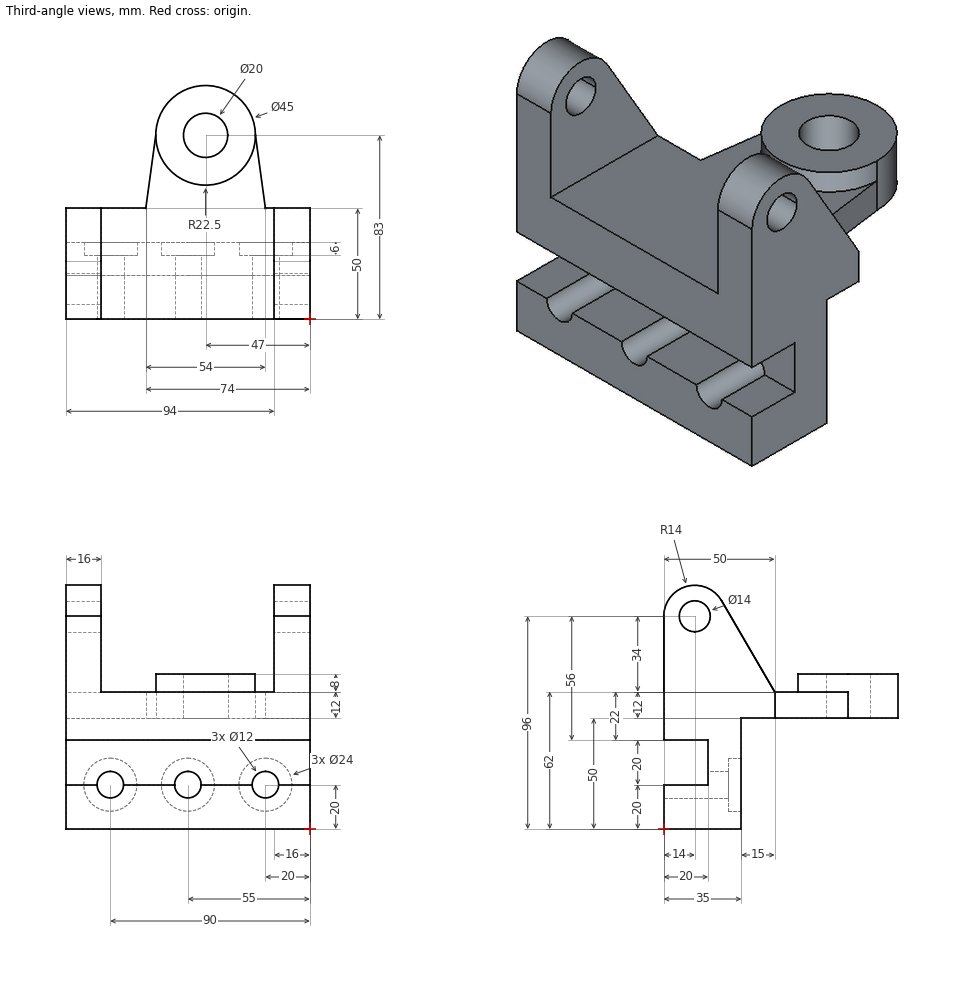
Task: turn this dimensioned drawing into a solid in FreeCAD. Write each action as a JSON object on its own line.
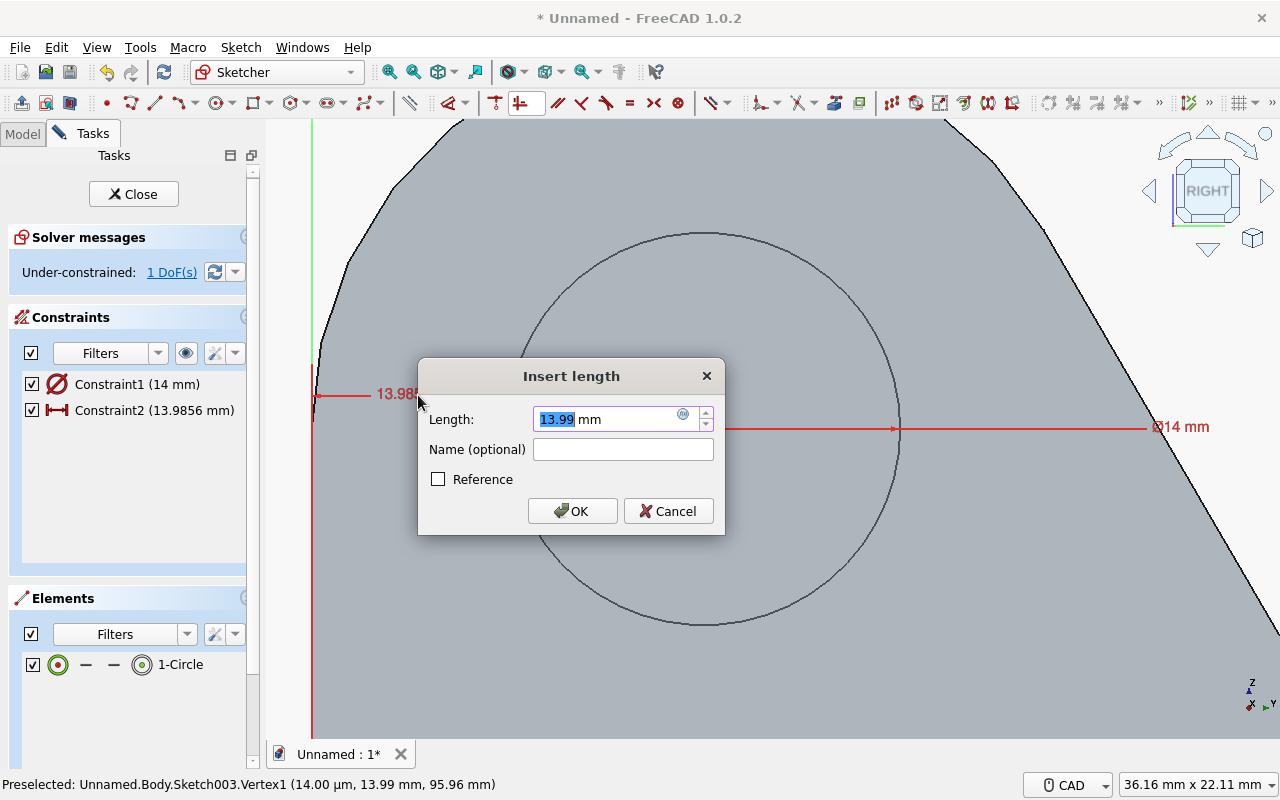
{"action": "type", "text": "14"}
{"action": "key", "text": "Return"}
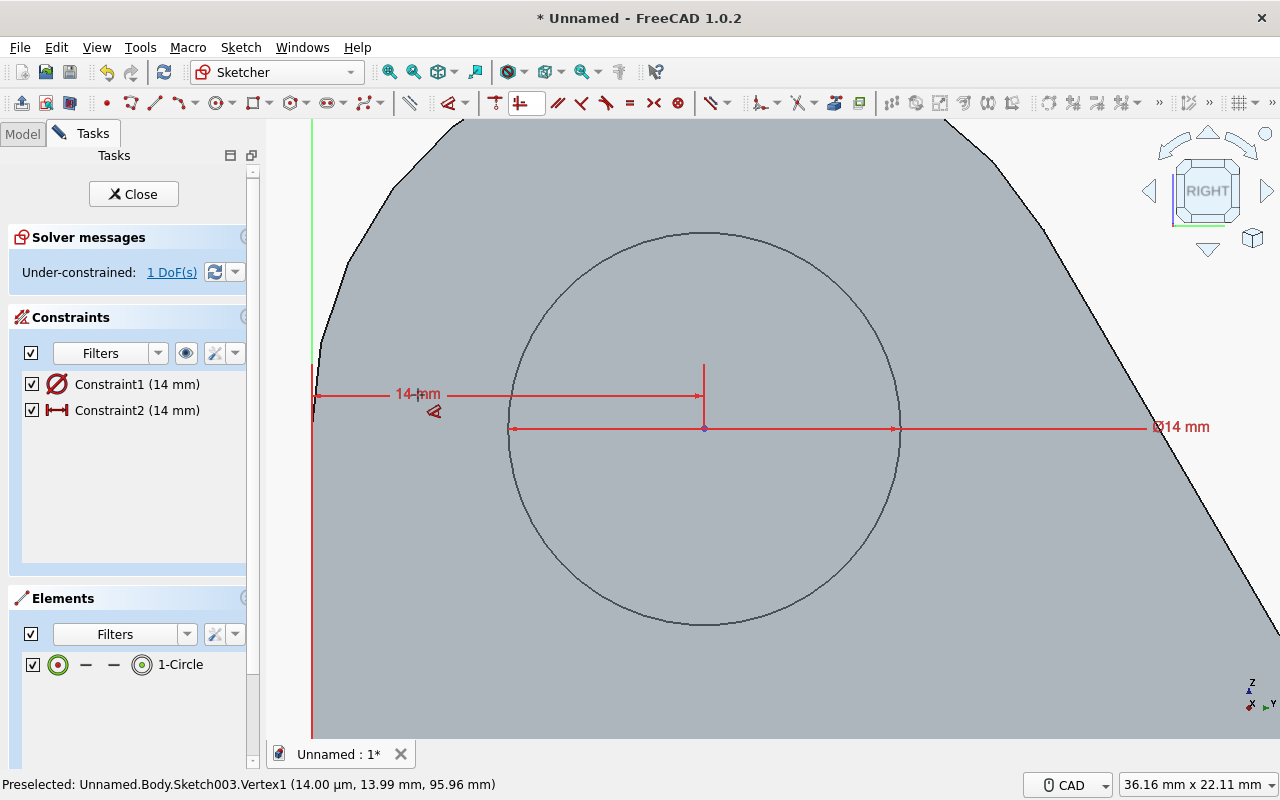
{"action": "left_click", "coordinate": [704, 429]}
{"action": "left_click", "coordinate": [738, 570]}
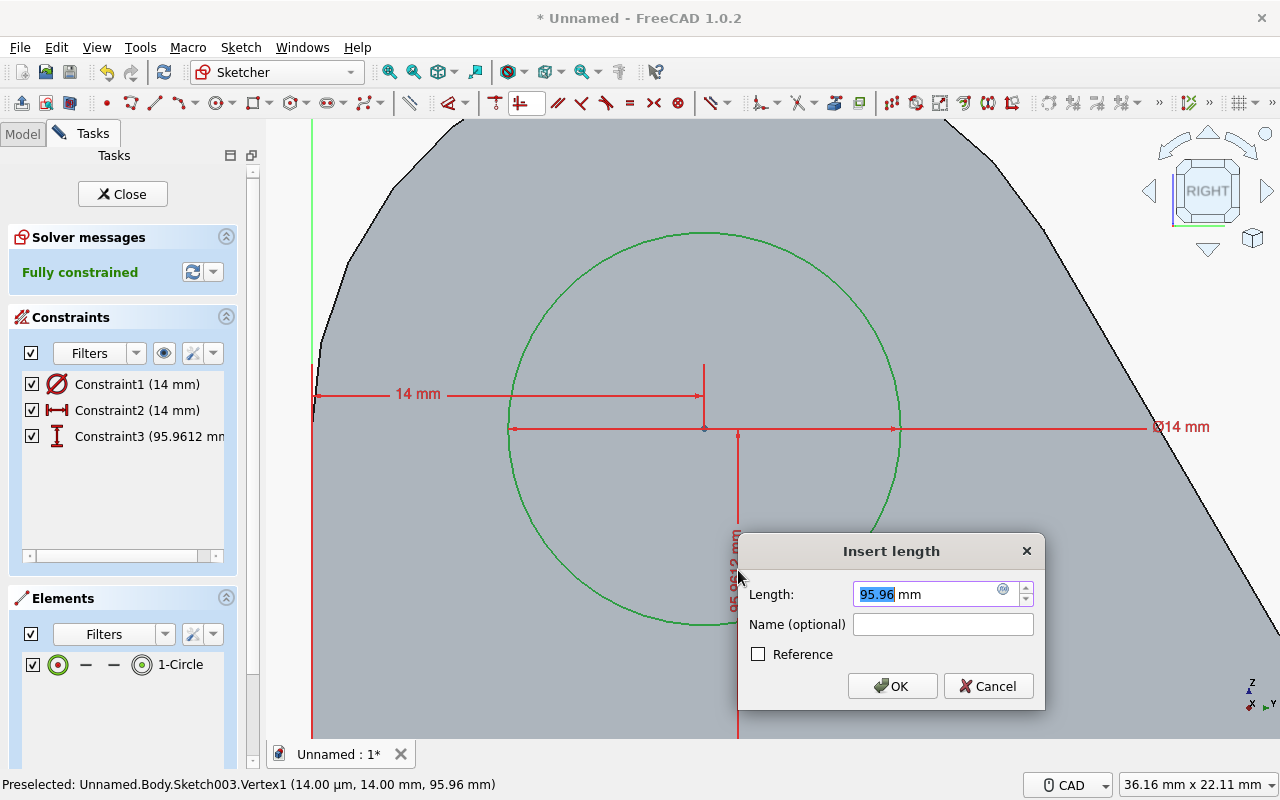
{"action": "type", "text": "96"}
{"action": "key", "text": "Return"}
{"action": "key", "text": "Escape"}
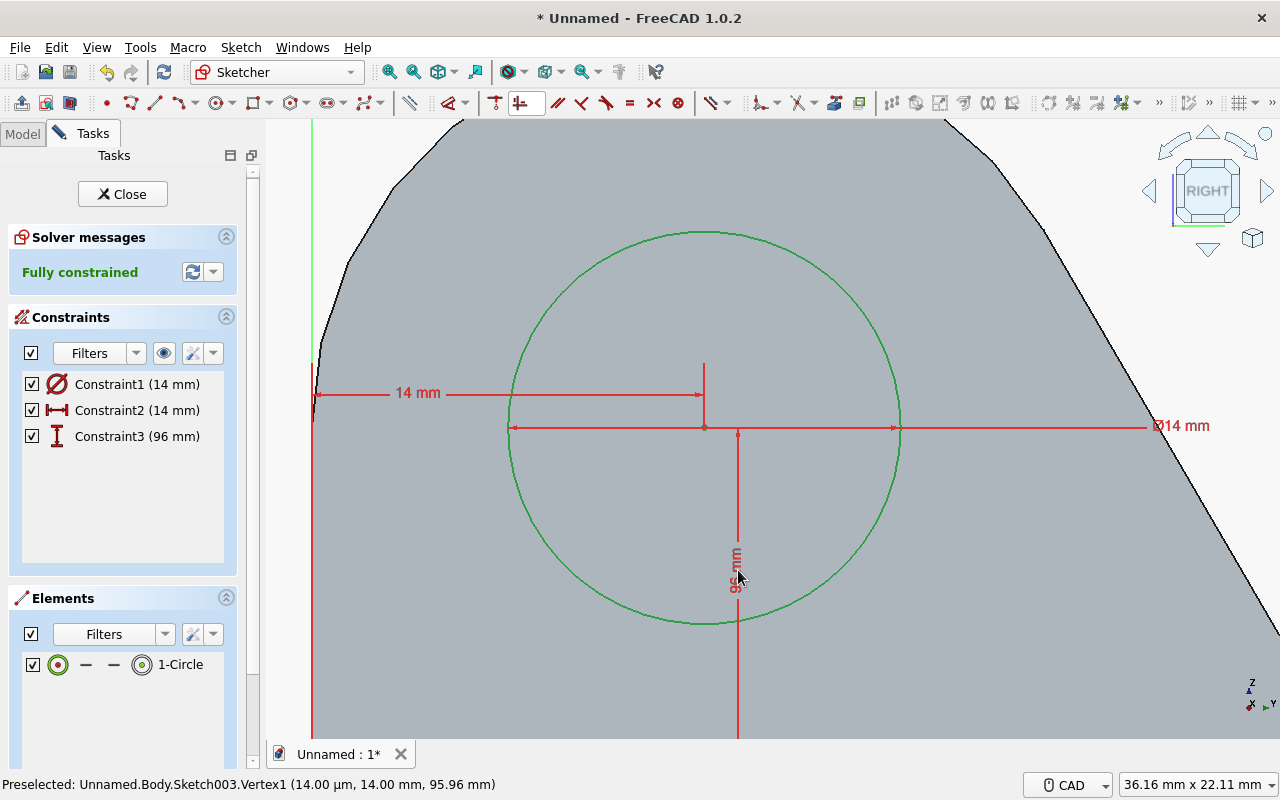
{"action": "left_click", "coordinate": [123, 194]}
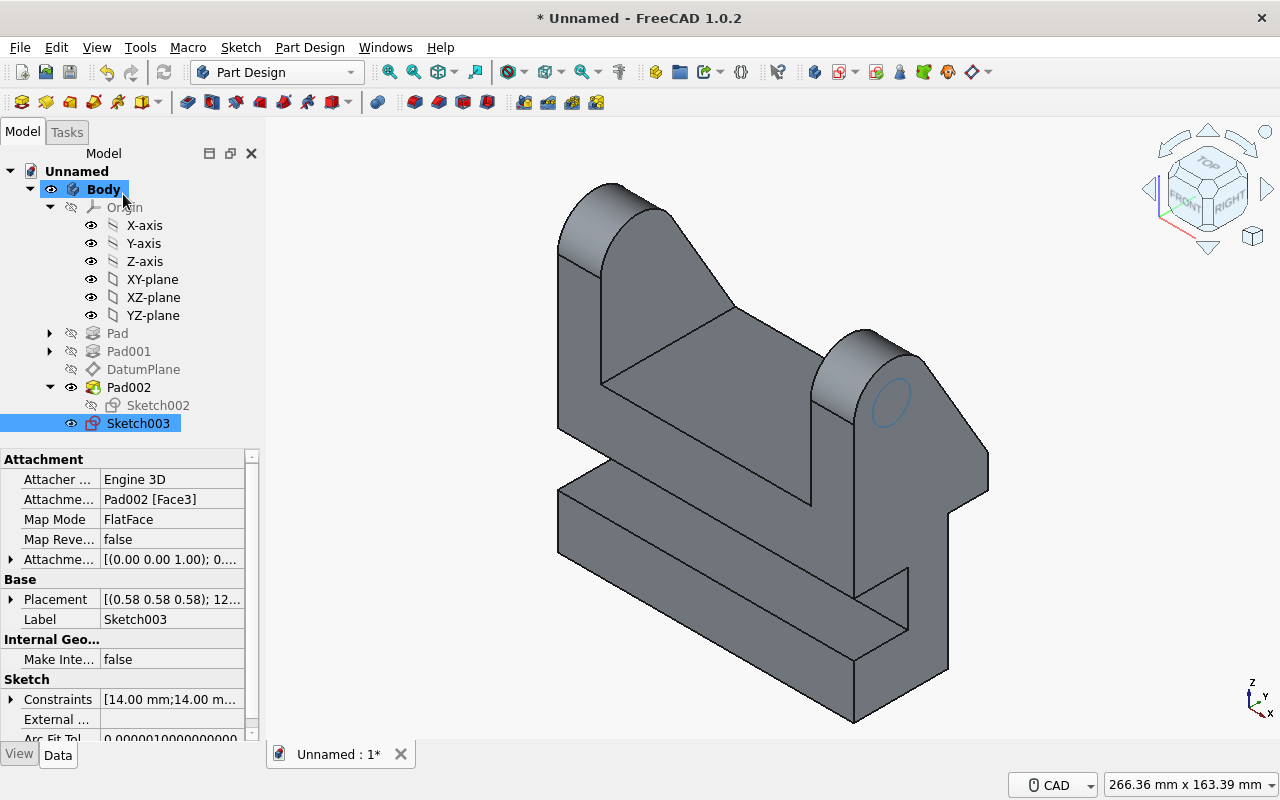
{"action": "left_click", "coordinate": [188, 102]}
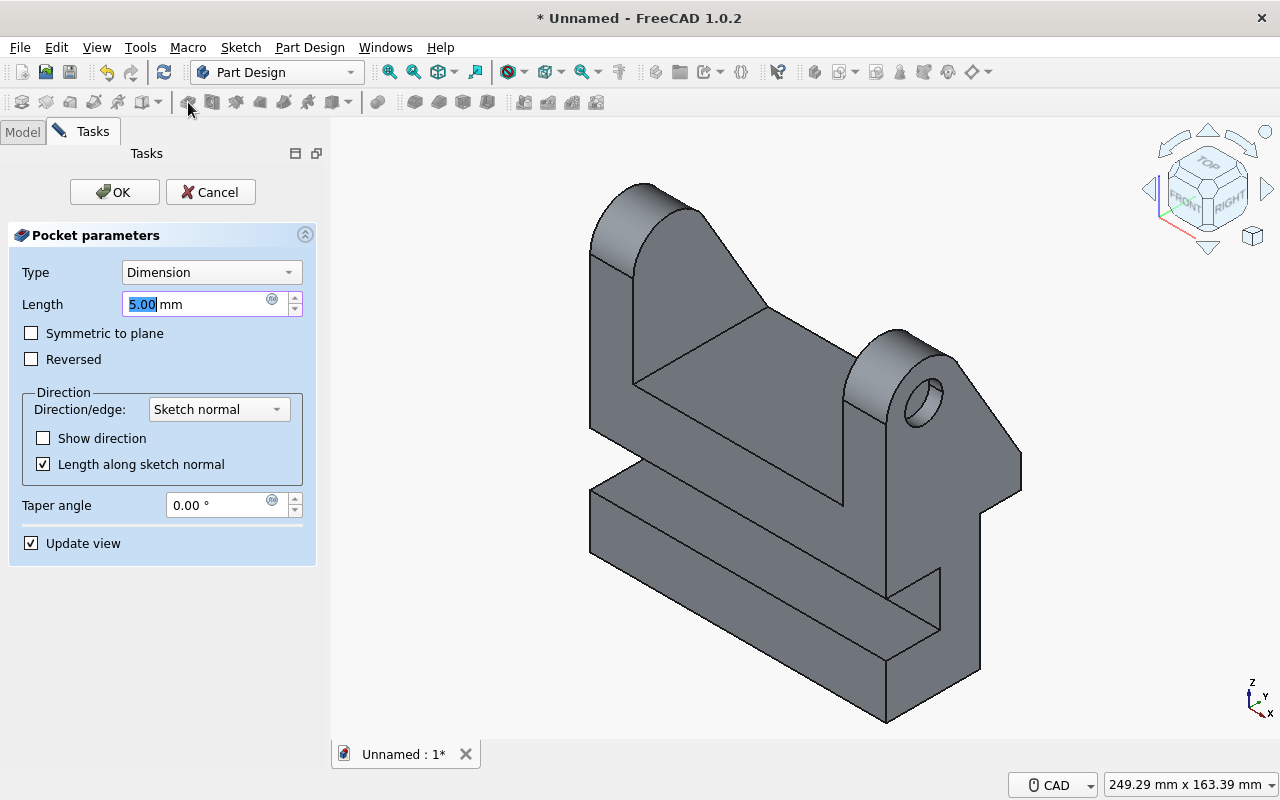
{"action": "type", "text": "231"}
{"action": "key", "text": "Tab"}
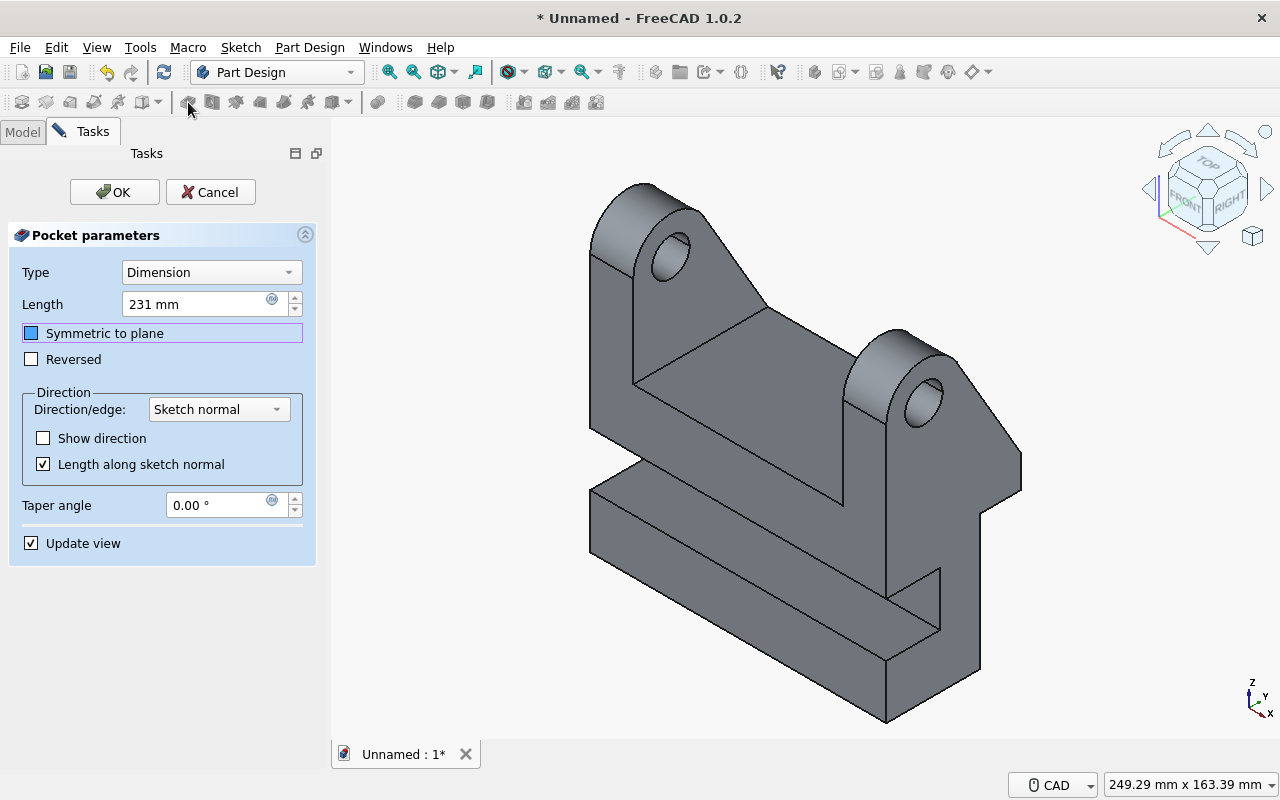
{"action": "left_click", "coordinate": [115, 192]}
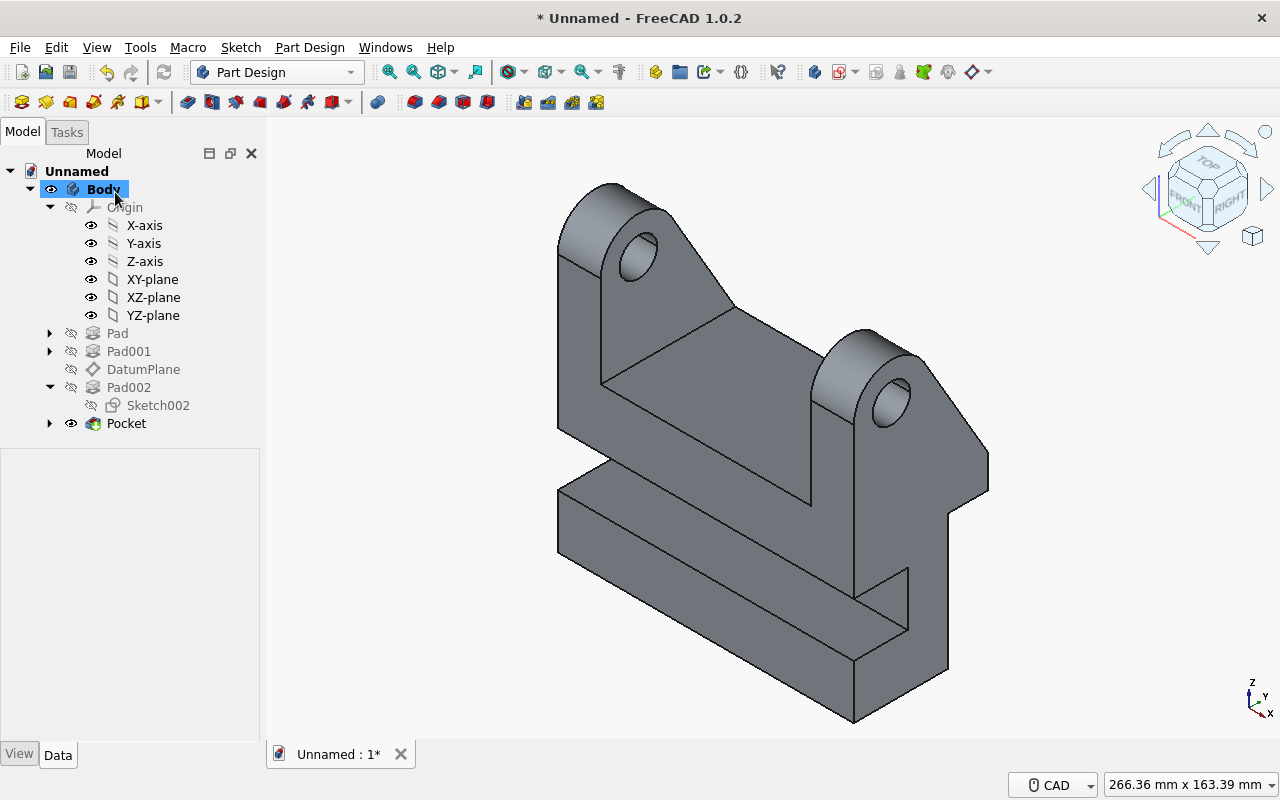
{"action": "left_click", "coordinate": [816, 72]}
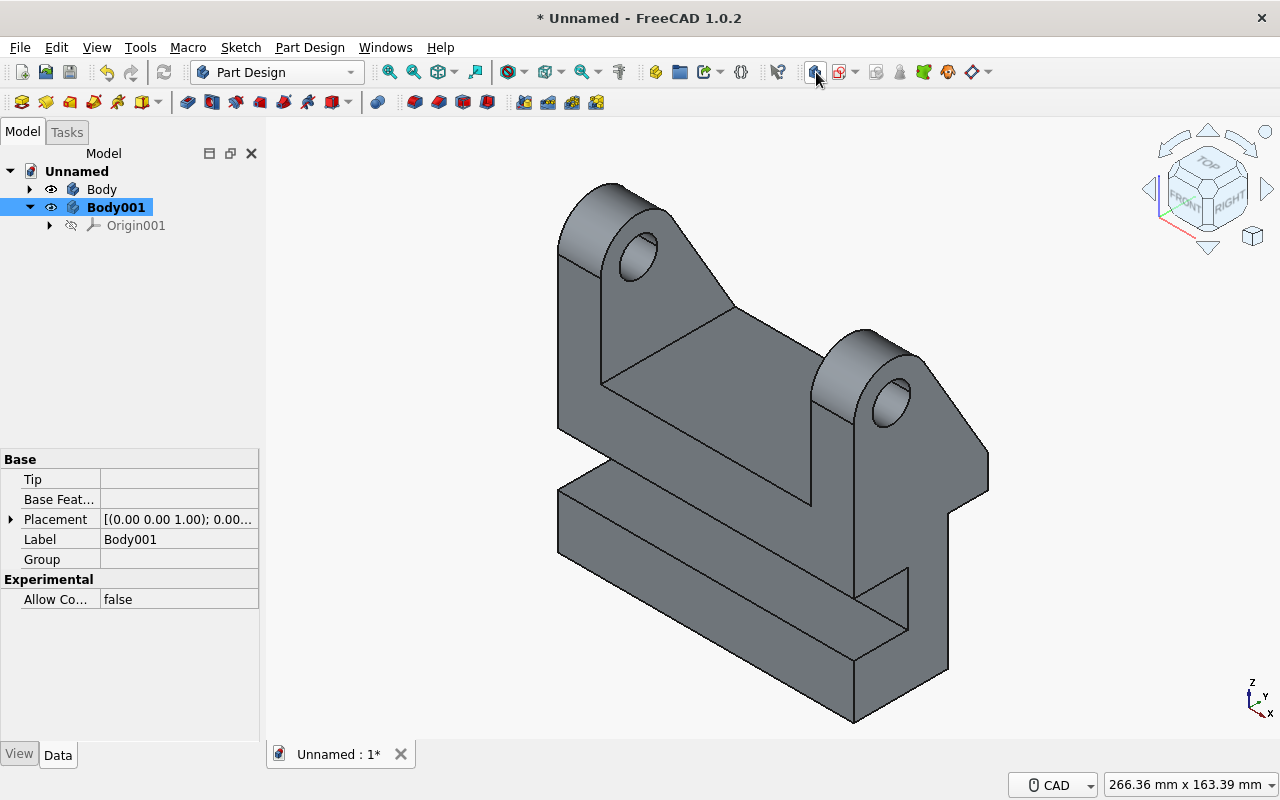
{"action": "left_click", "coordinate": [50, 225]}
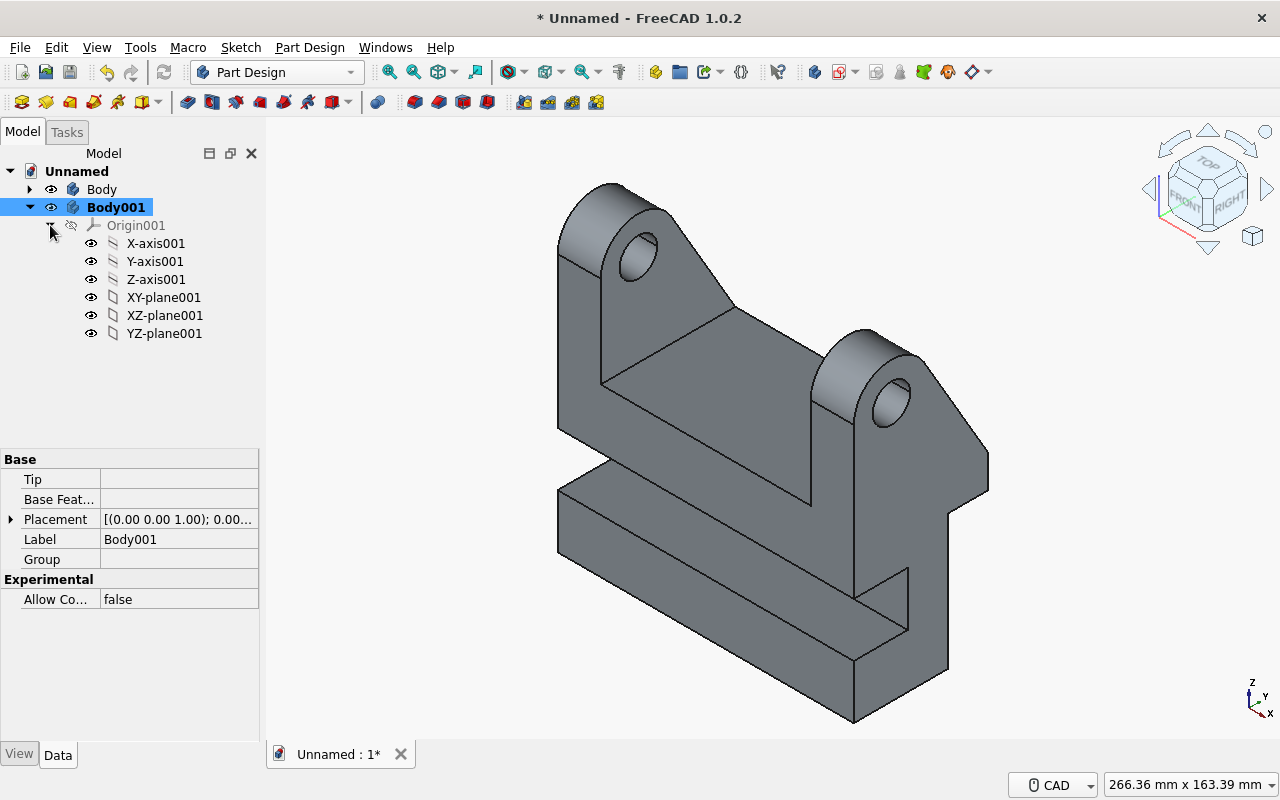
{"action": "left_click", "coordinate": [136, 297]}